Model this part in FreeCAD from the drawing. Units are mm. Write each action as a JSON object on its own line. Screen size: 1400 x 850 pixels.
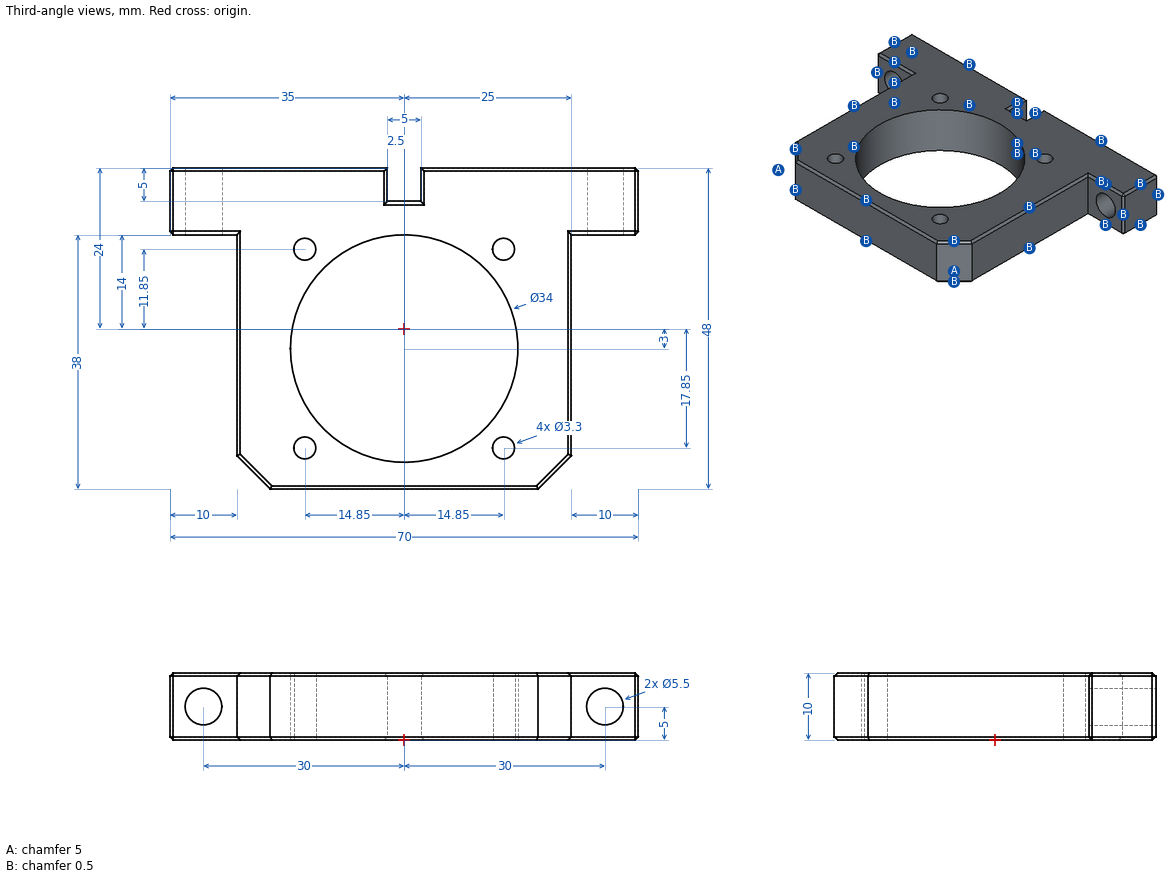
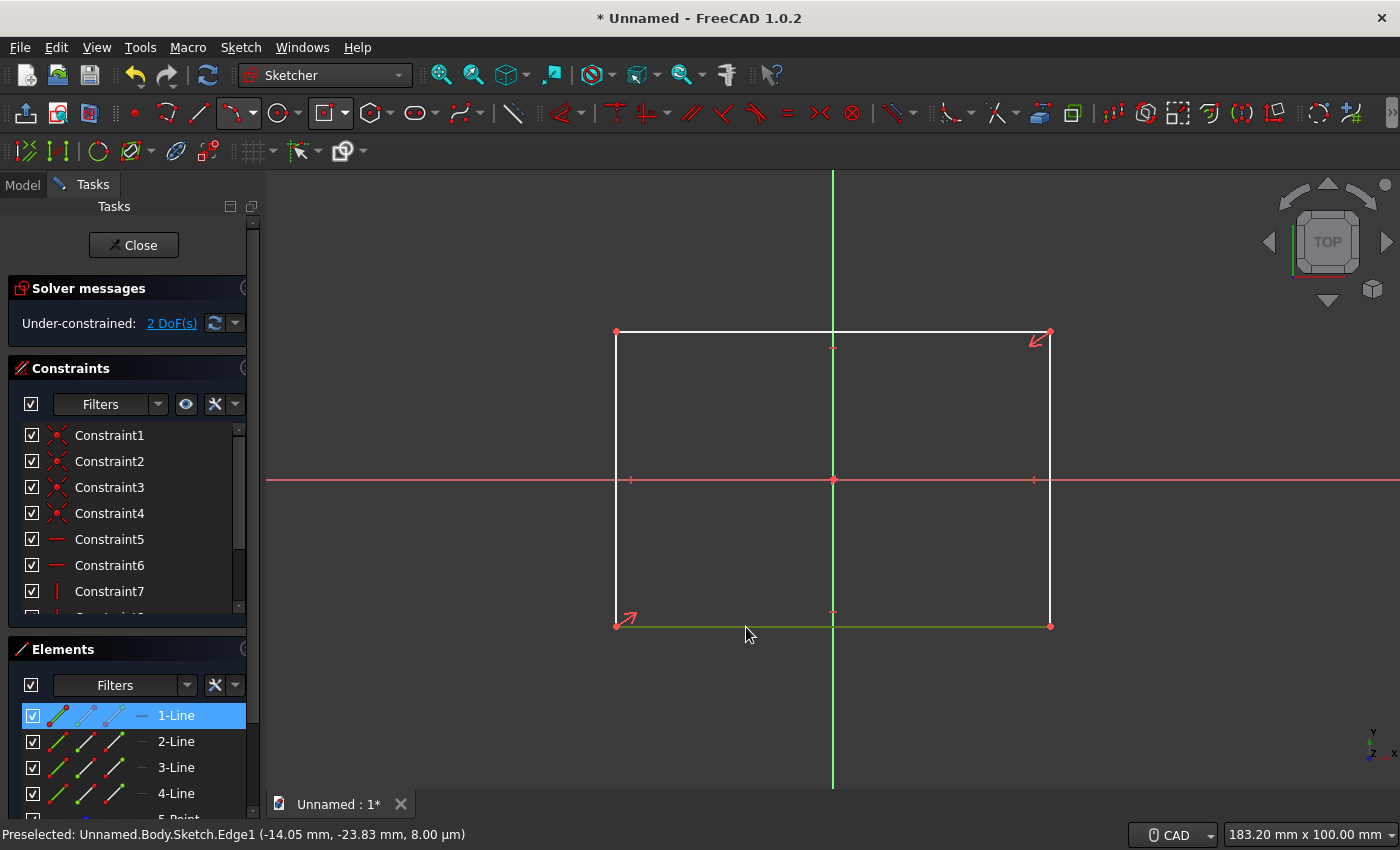
{"action": "key", "text": "l"}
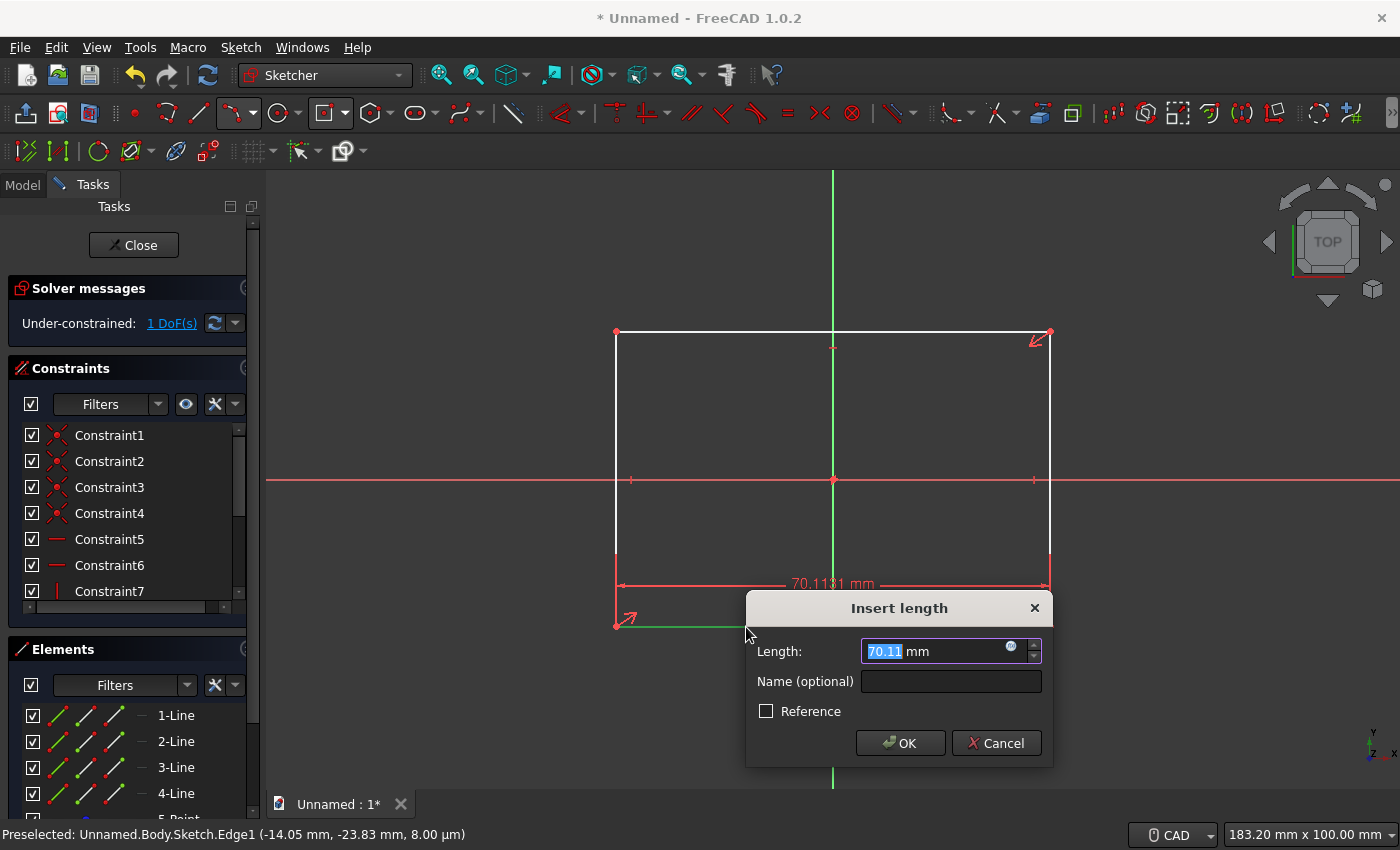
{"action": "type", "text": "70"}
{"action": "key", "text": "Return"}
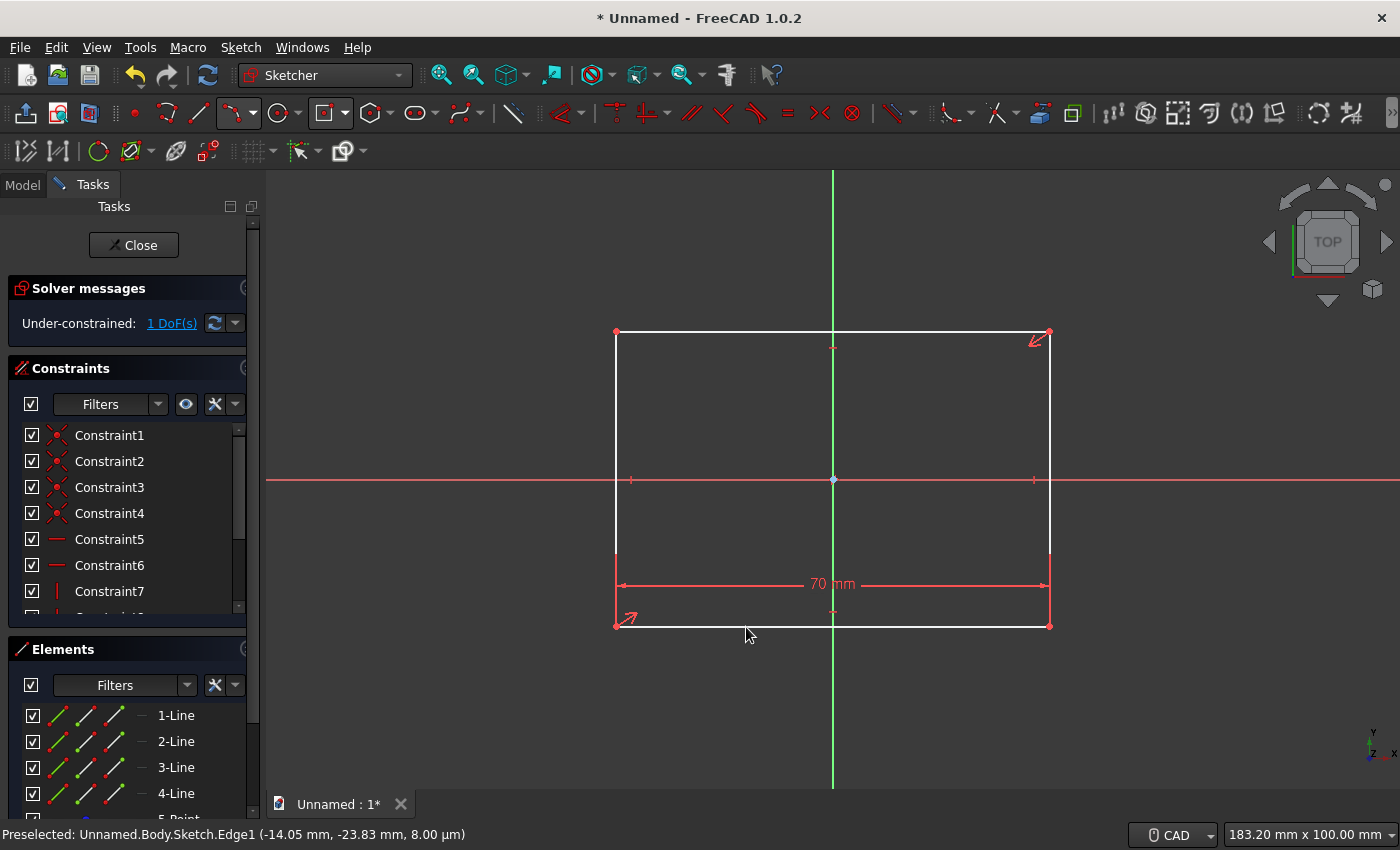
{"action": "left_click", "coordinate": [1050, 538]}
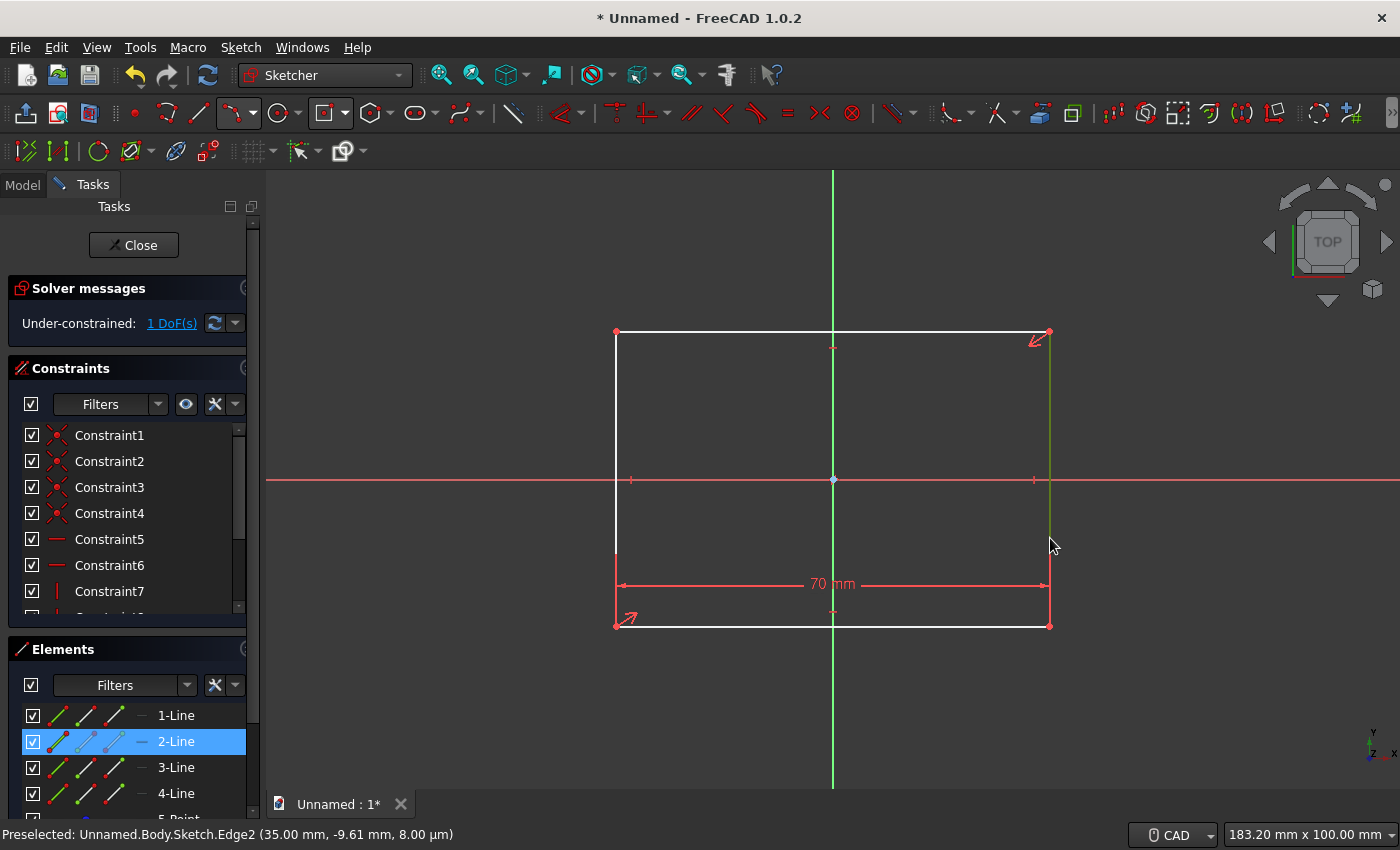
{"action": "left_click", "coordinate": [584, 114]}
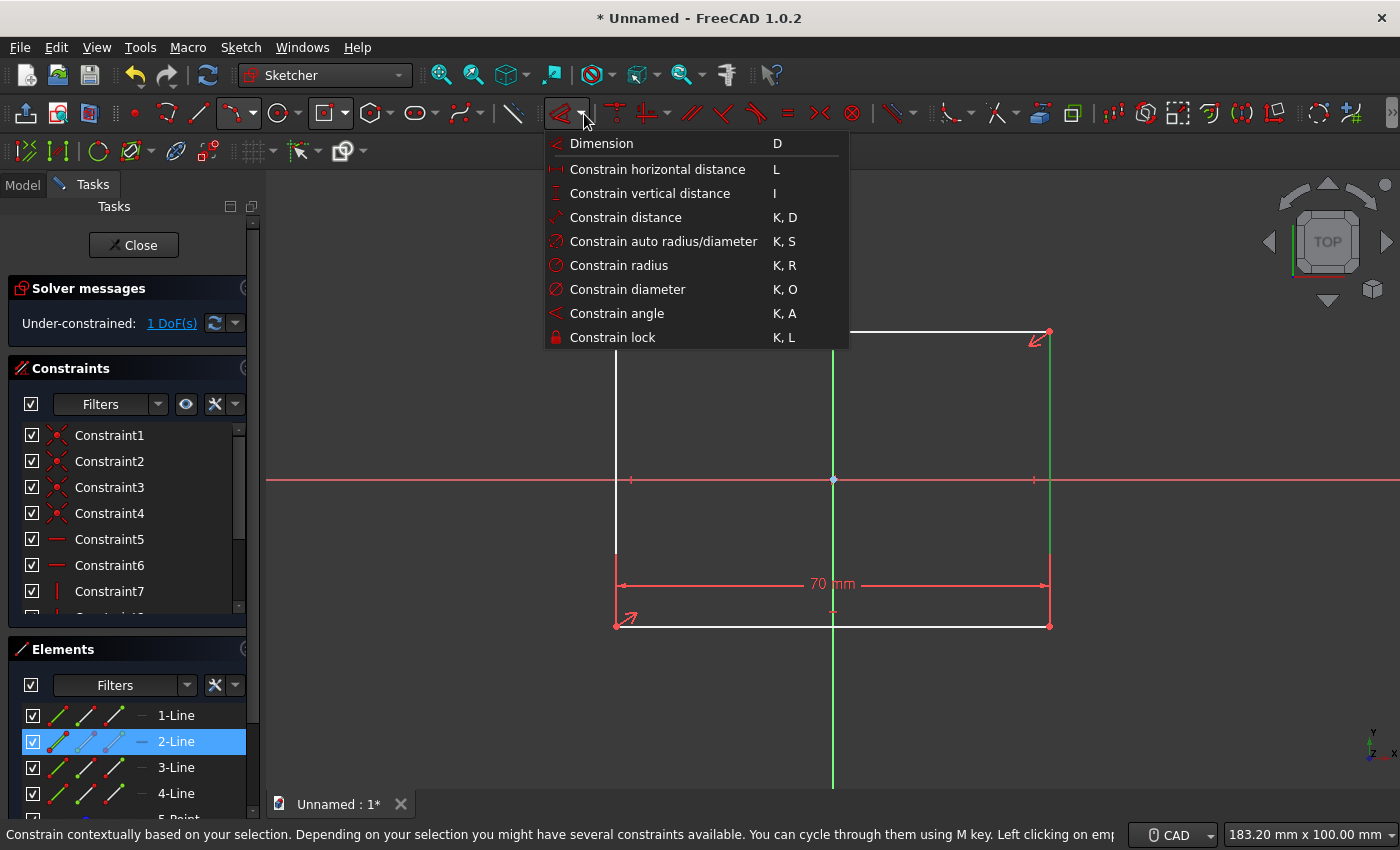
{"action": "left_click", "coordinate": [697, 193]}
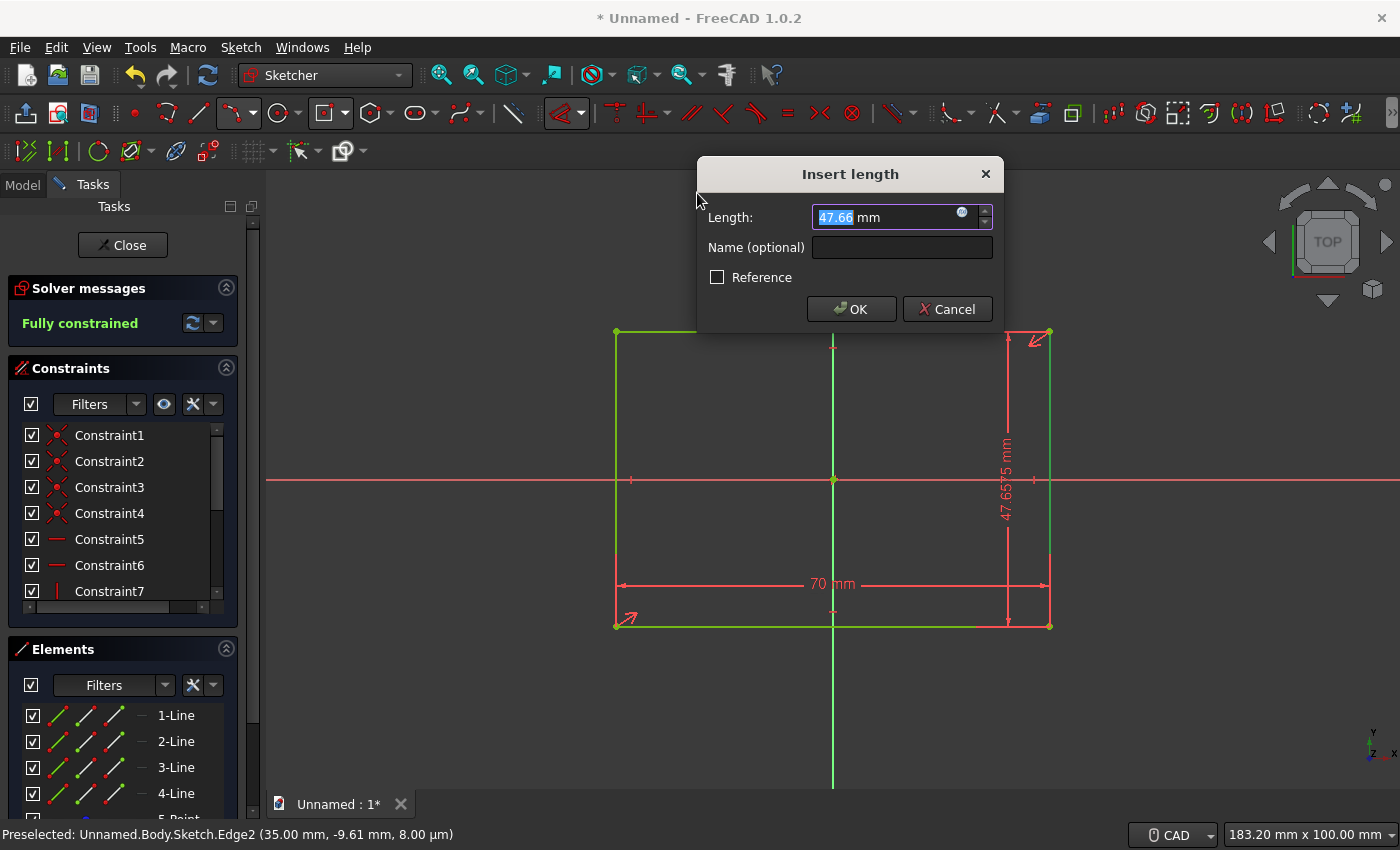
{"action": "type", "text": "48"}
{"action": "key", "text": "Return"}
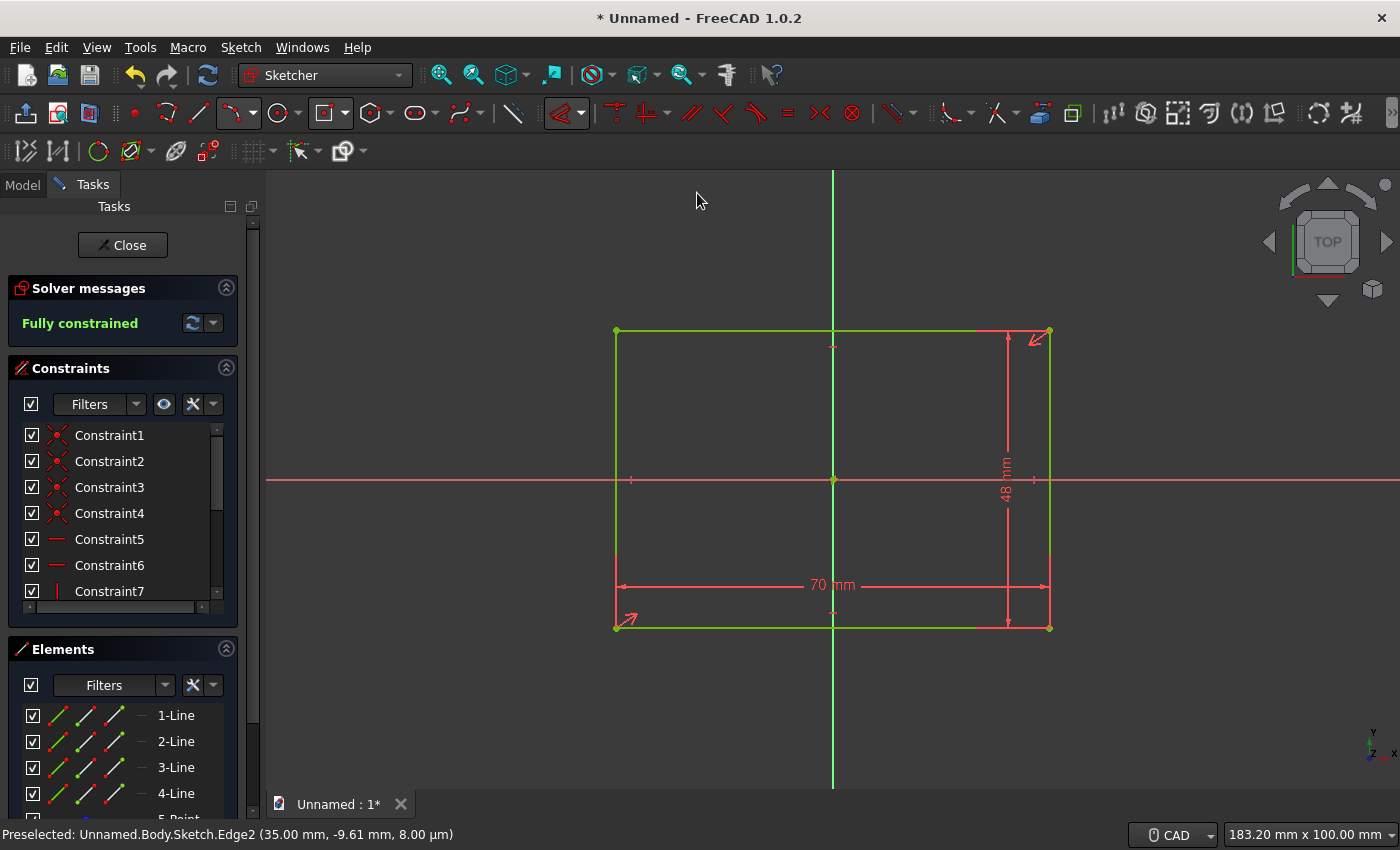
{"action": "left_click", "coordinate": [123, 245]}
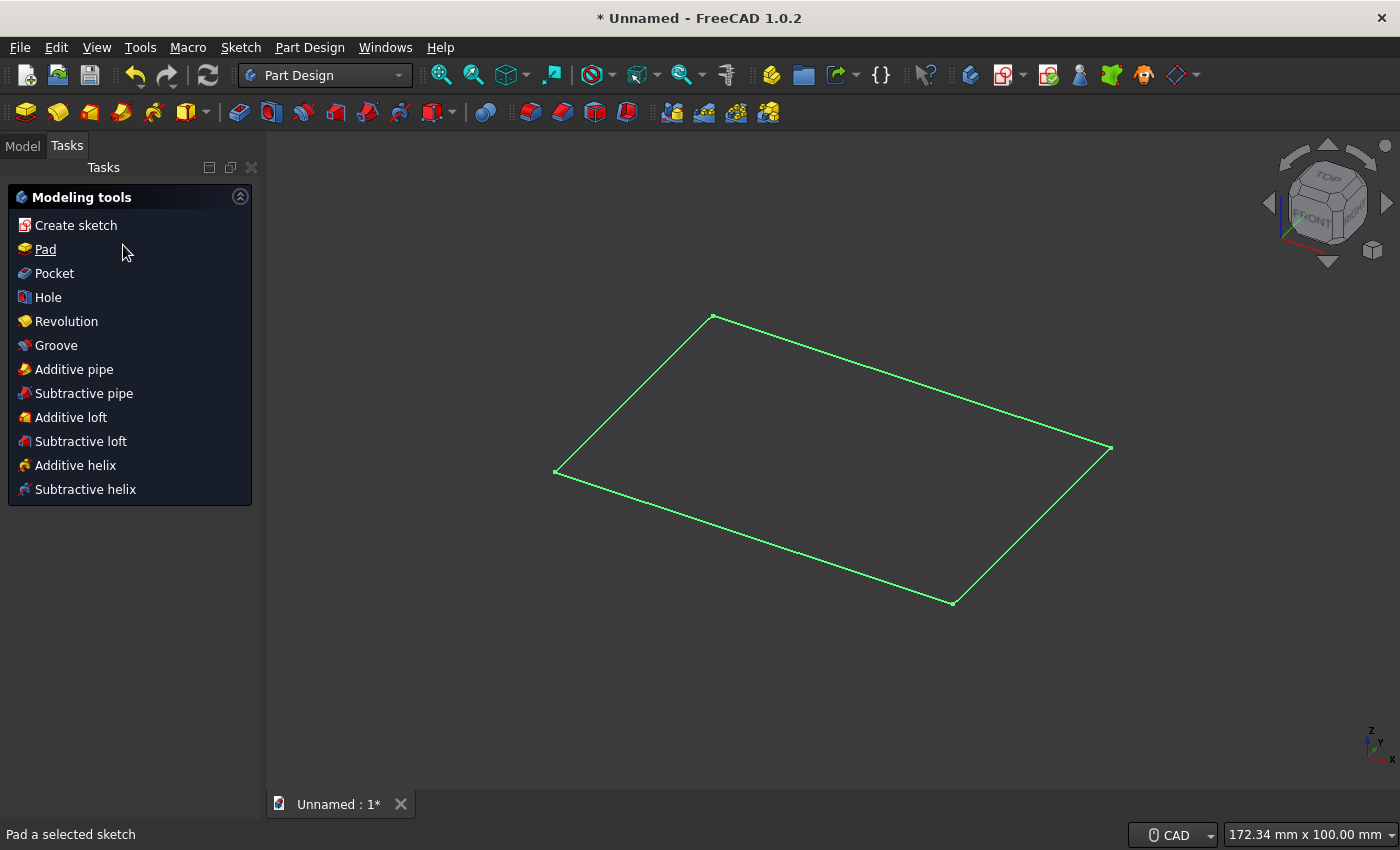
{"action": "left_click", "coordinate": [26, 112]}